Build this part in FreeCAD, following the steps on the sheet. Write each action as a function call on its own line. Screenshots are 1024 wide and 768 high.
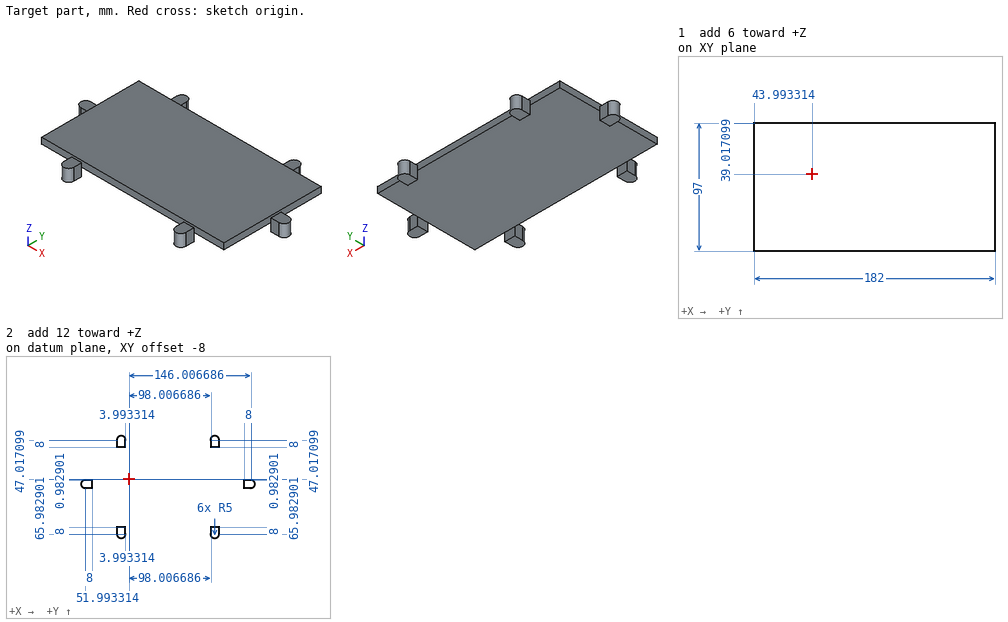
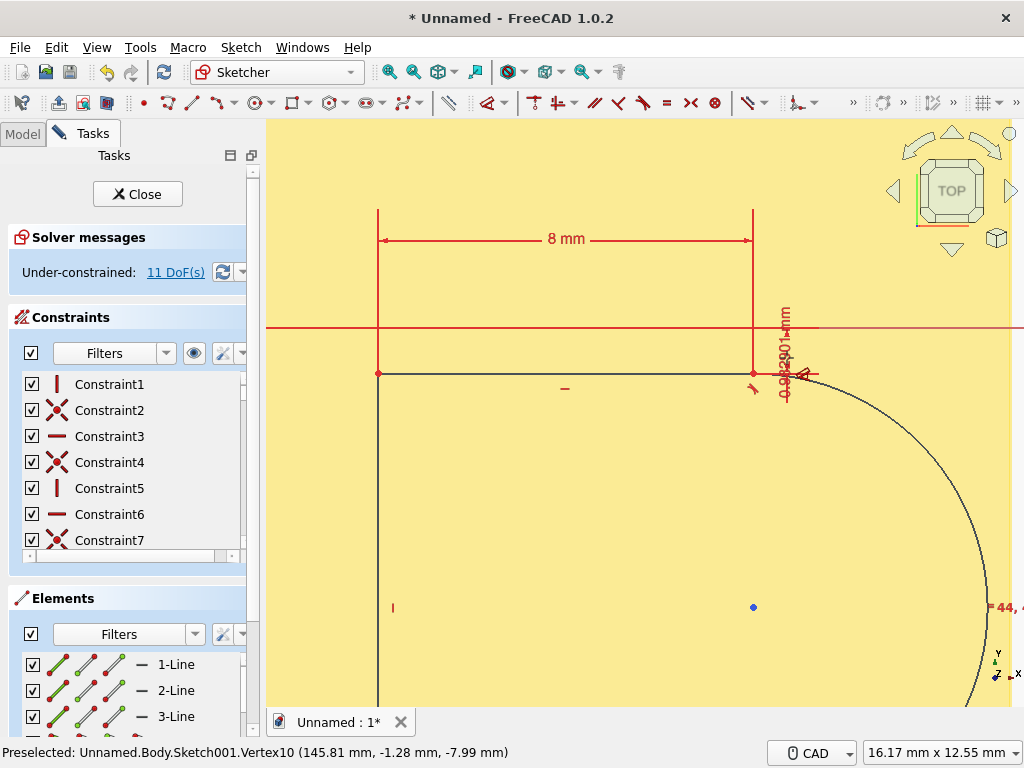
scroll(810, 394, down, 15)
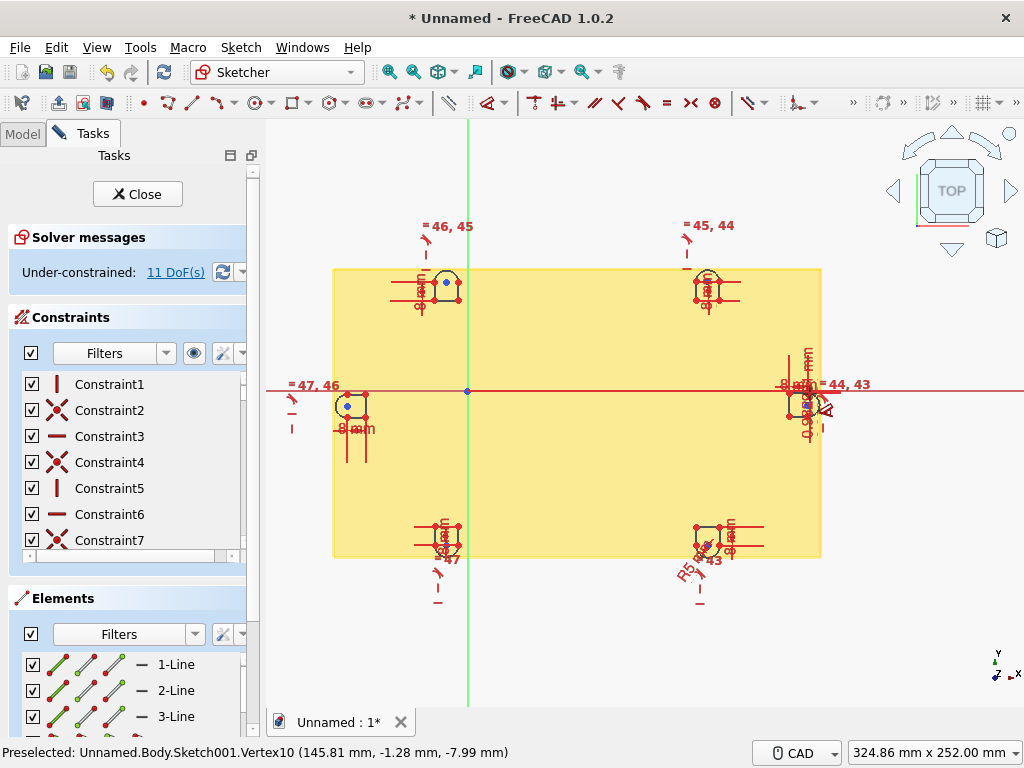
scroll(458, 301, up, 8)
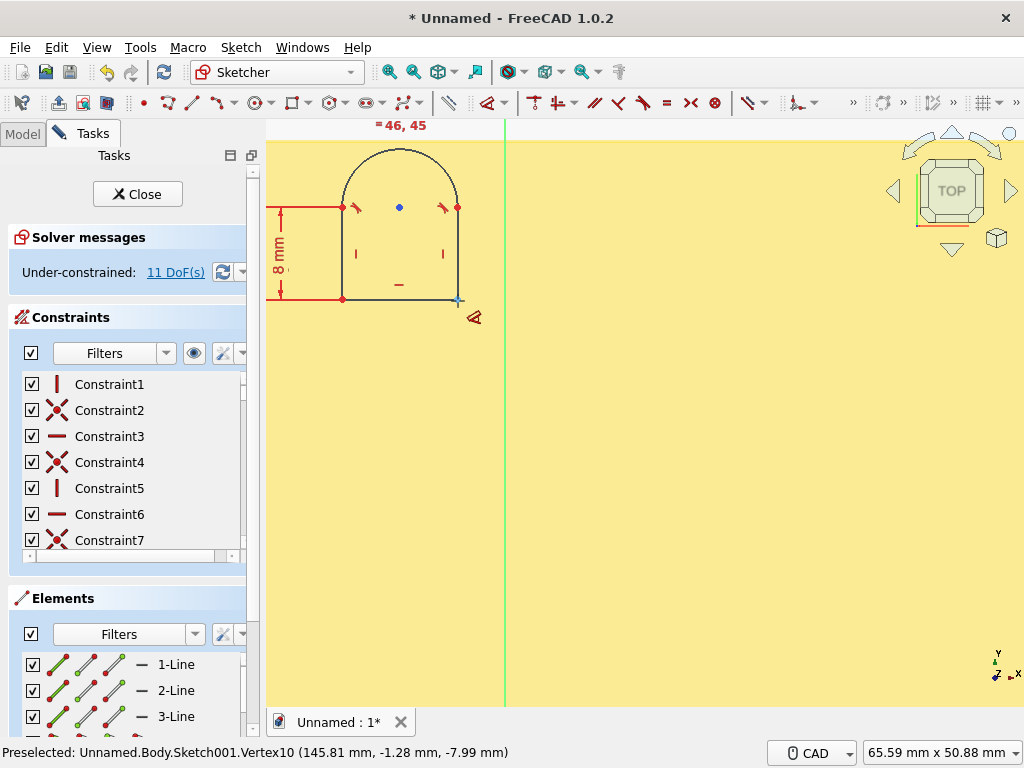
click(458, 300)
click(481, 266)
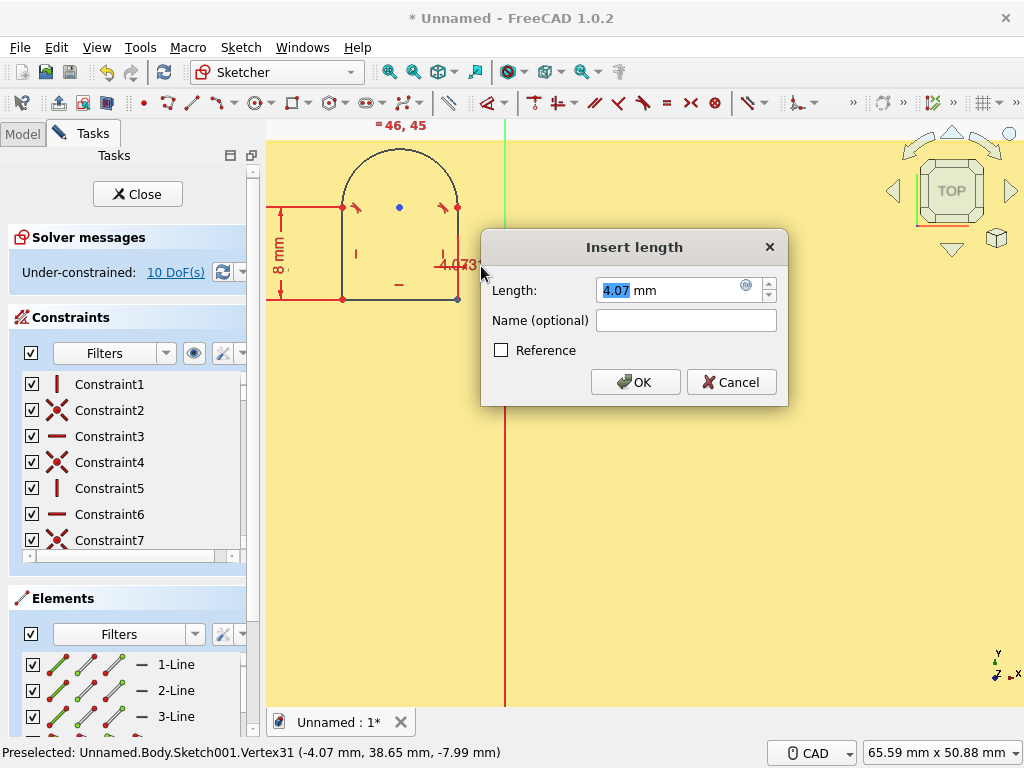
text(3.993314)
key(Return)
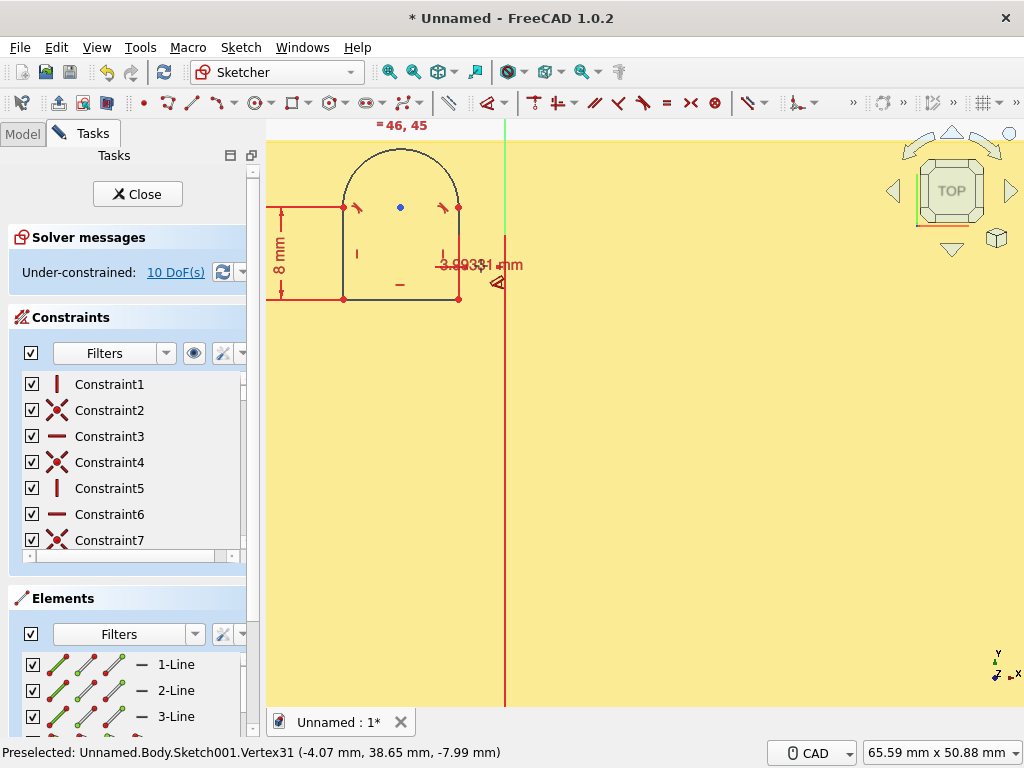
scroll(483, 325, down, 9)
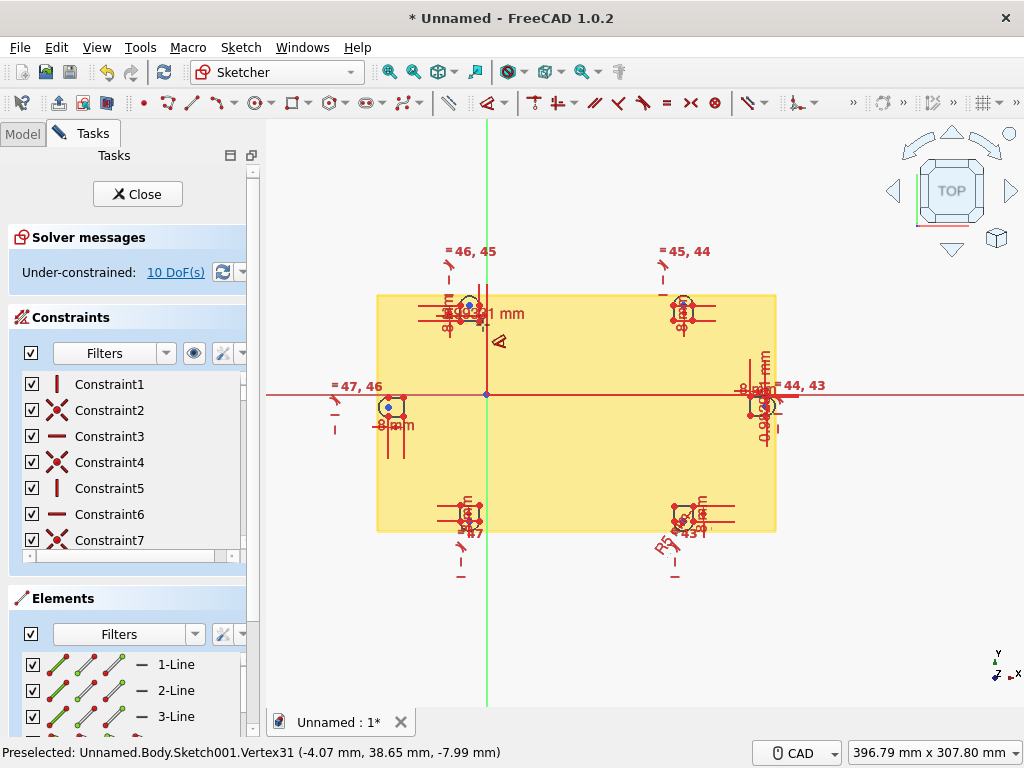
scroll(404, 398, up, 16)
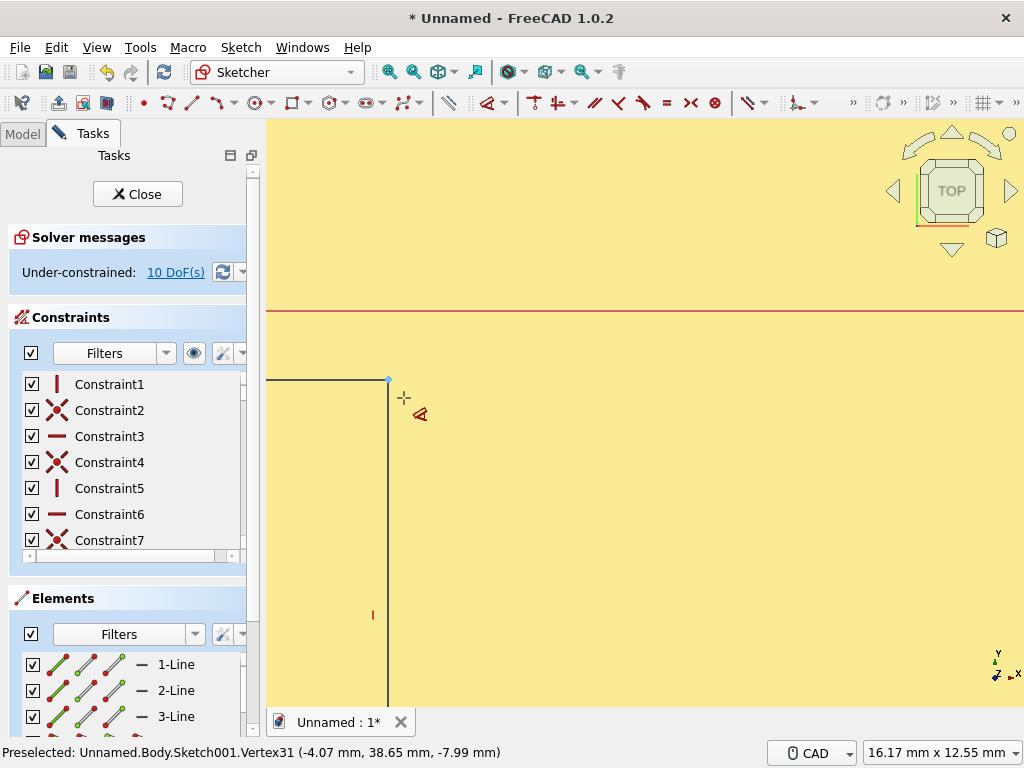
click(388, 380)
click(354, 346)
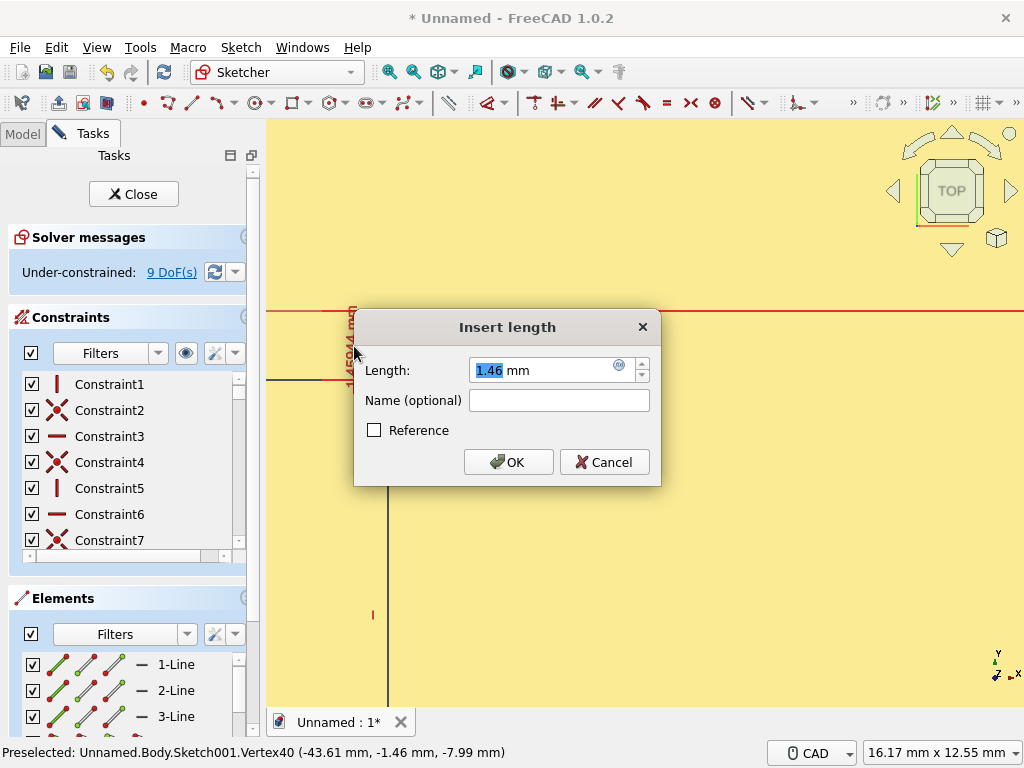
text(0.982901)
key(Return)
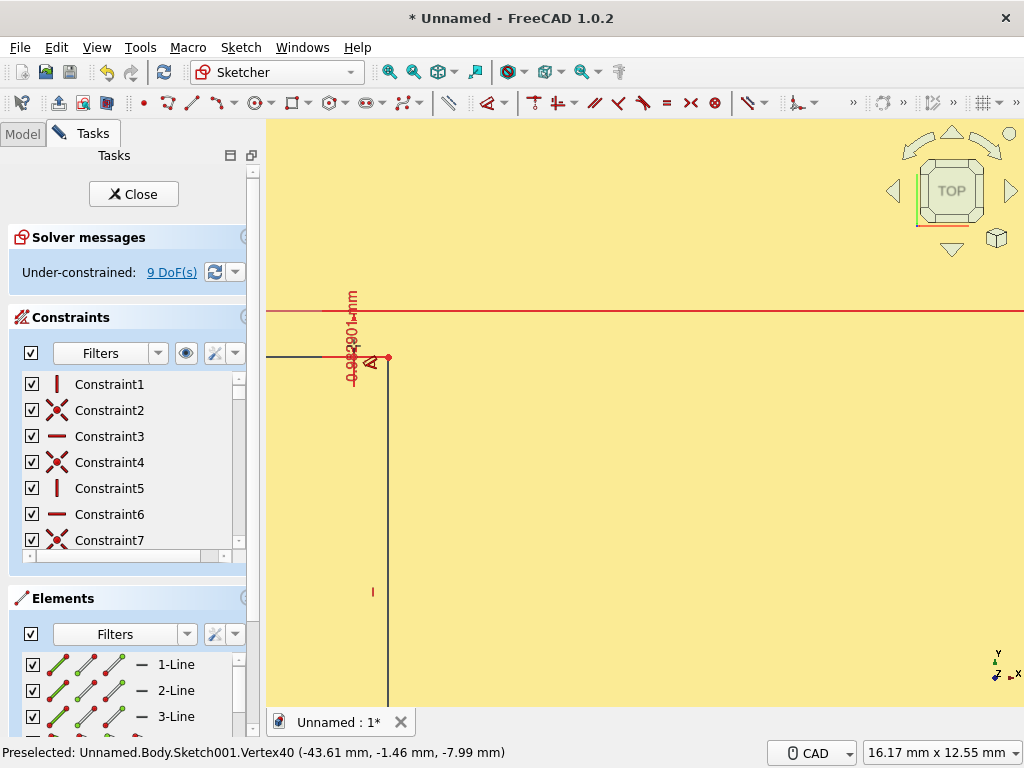
scroll(364, 395, down, 15)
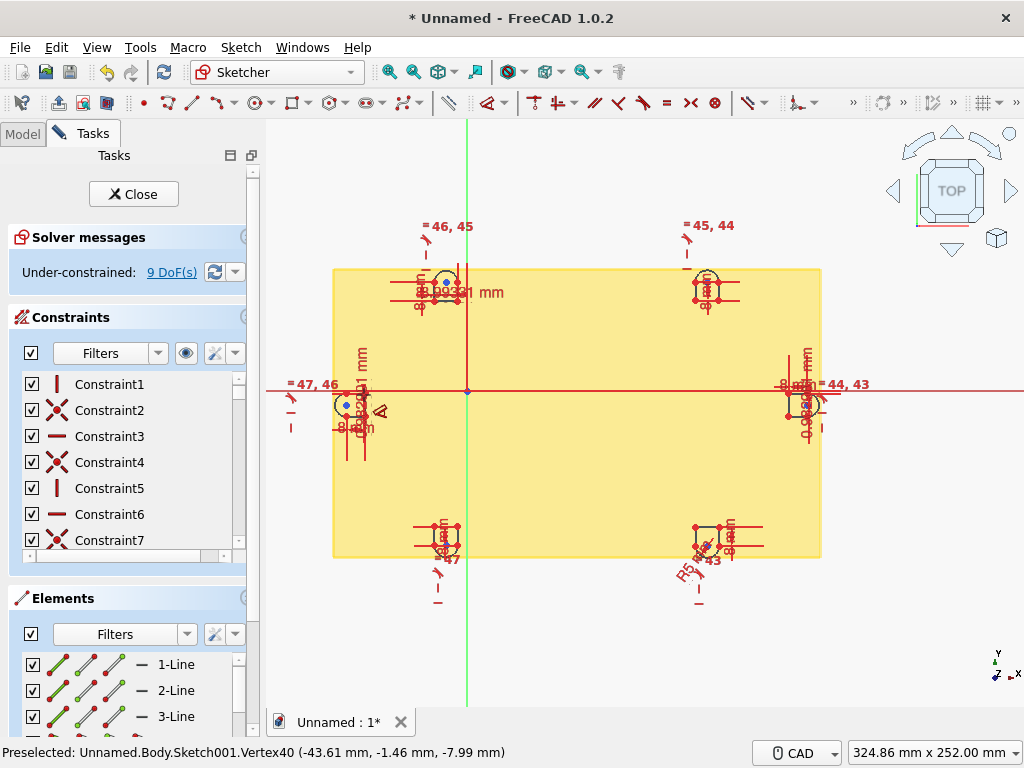
scroll(458, 546, up, 8)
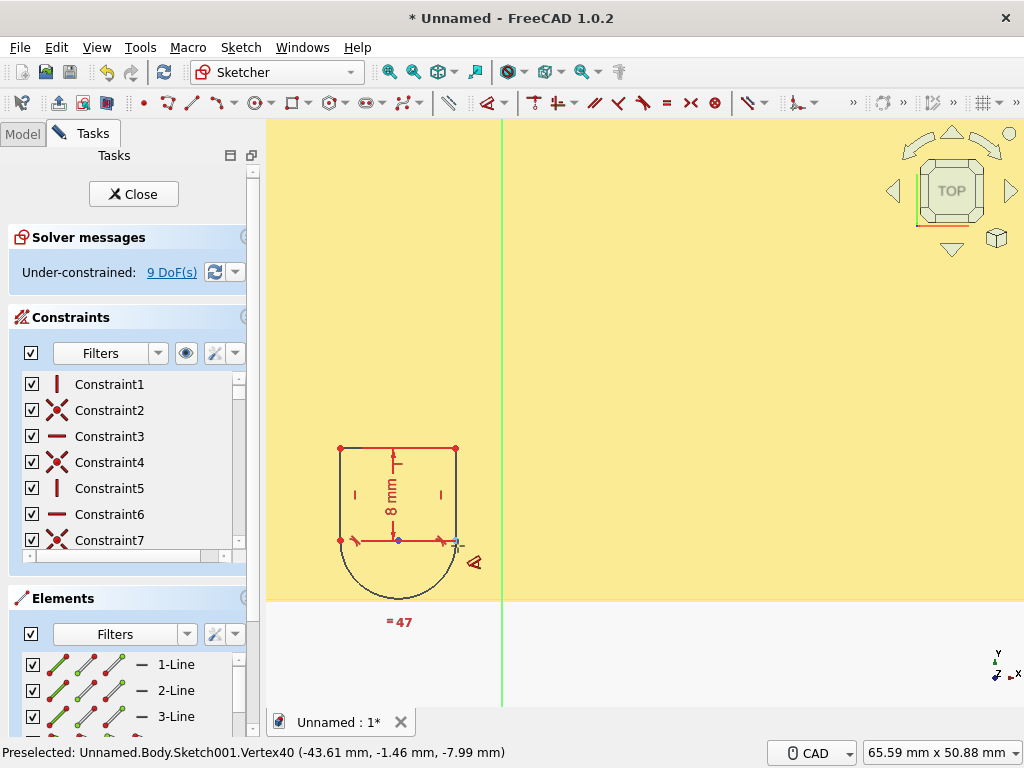
click(456, 541)
click(479, 575)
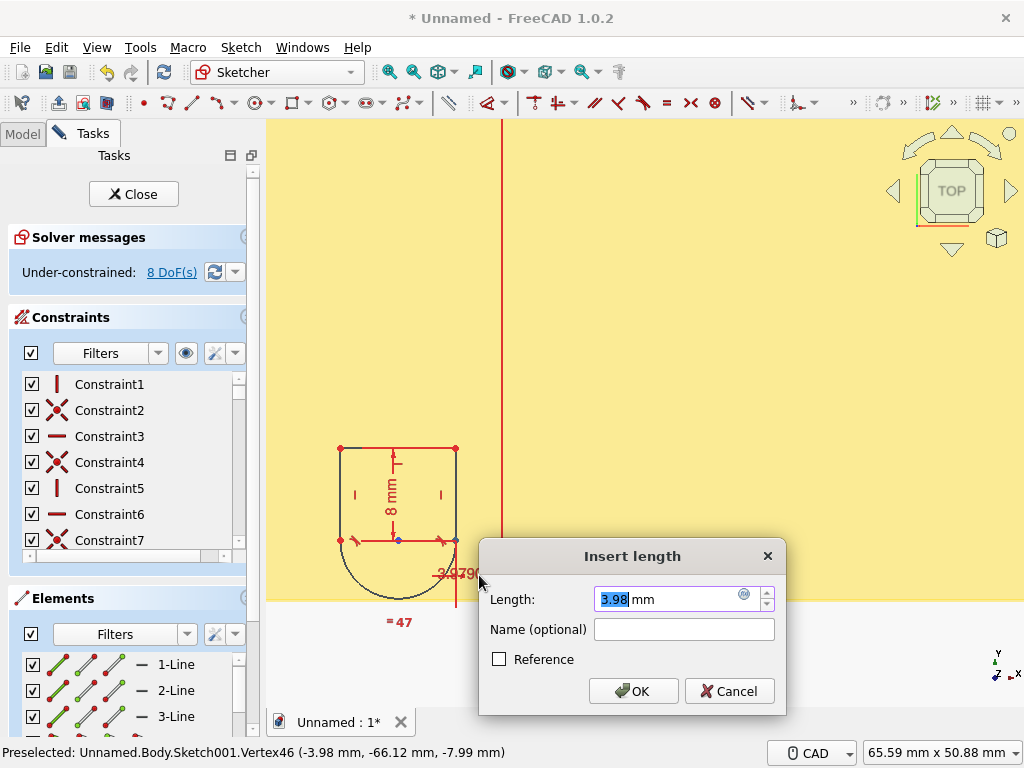
text(3.993314)
key(Return)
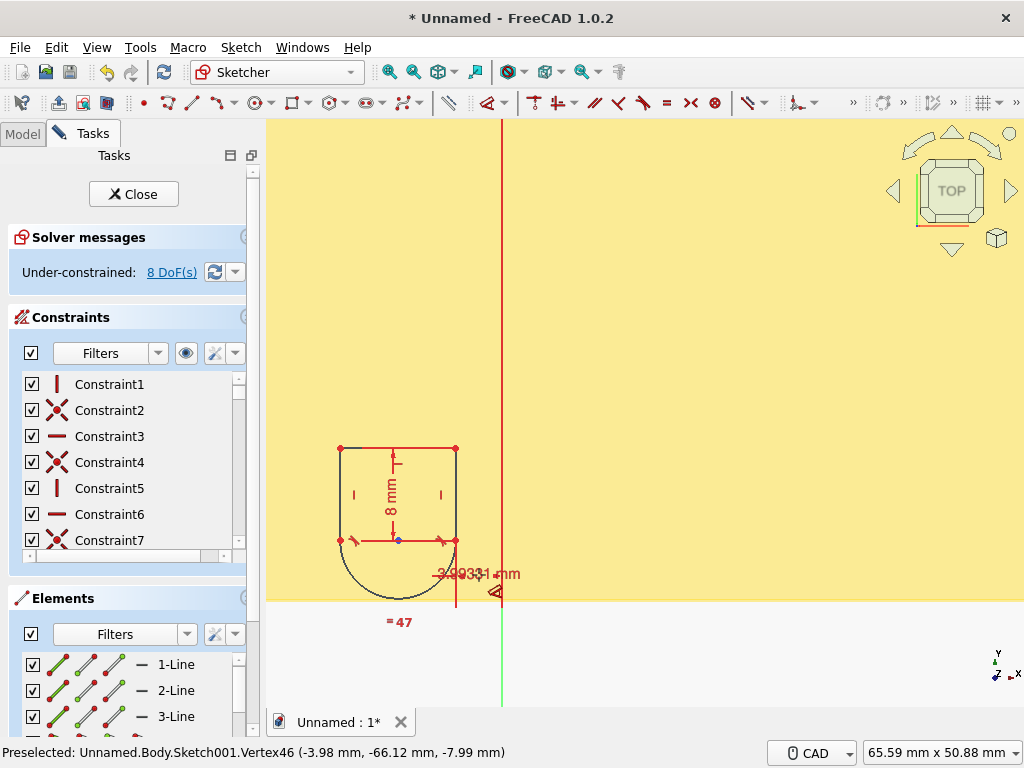
scroll(484, 517, down, 9)